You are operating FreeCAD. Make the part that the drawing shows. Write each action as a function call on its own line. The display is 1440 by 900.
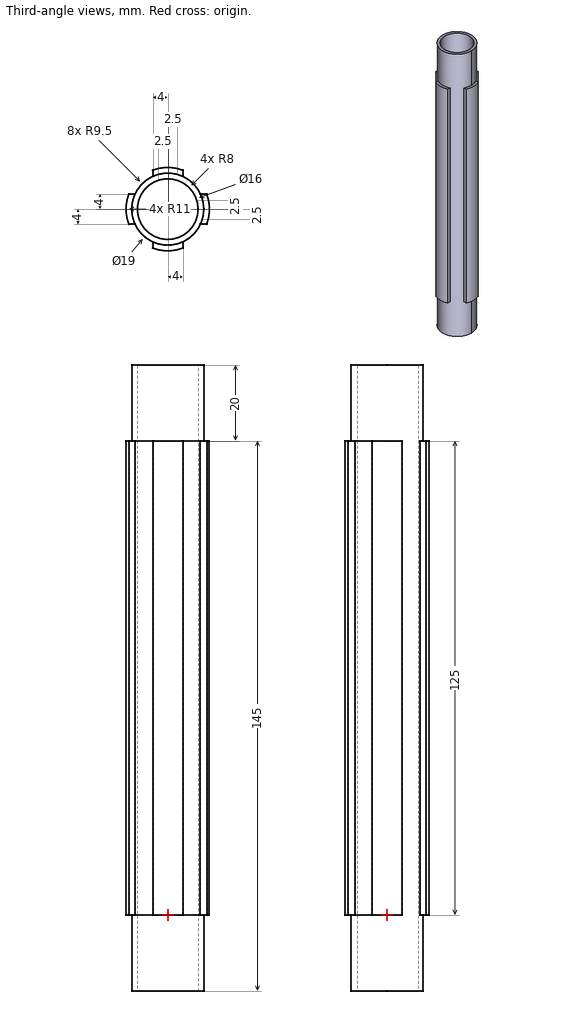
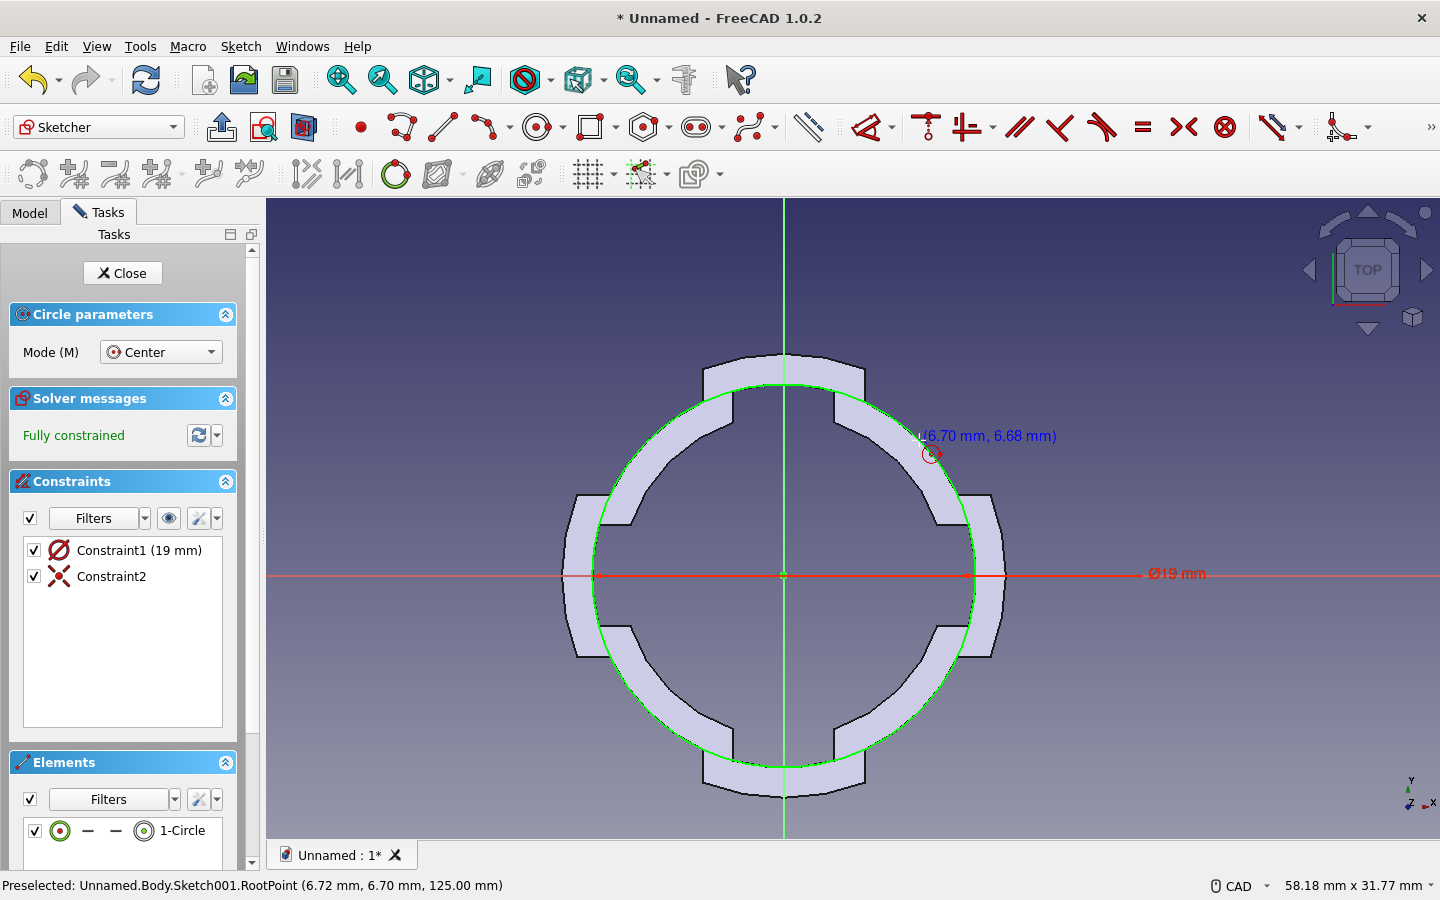
click(784, 576)
move(898, 462)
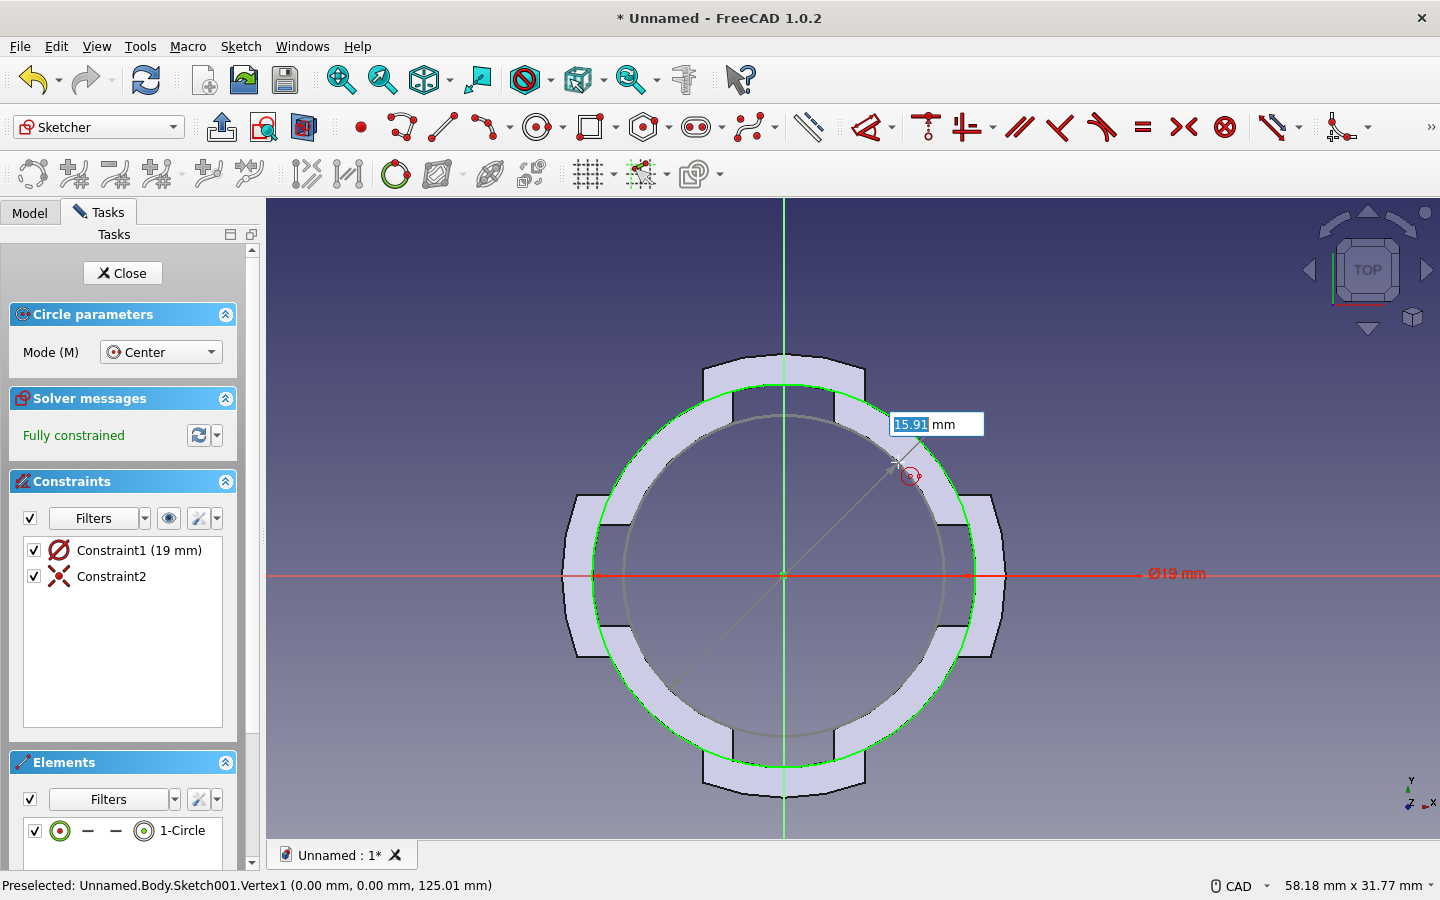
text(16)
key(Return)
key(Escape)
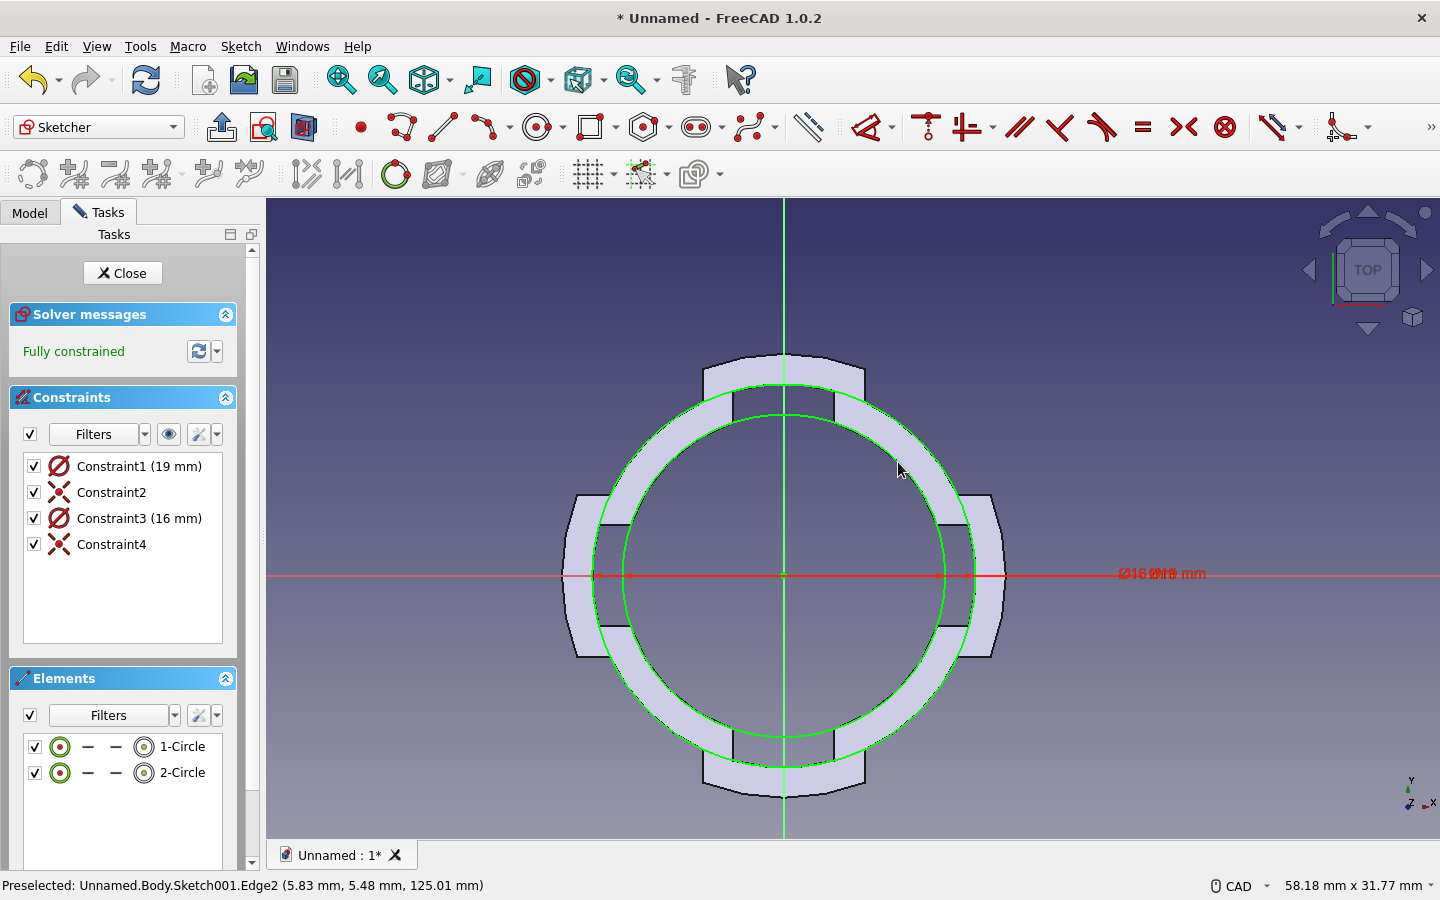
click(123, 273)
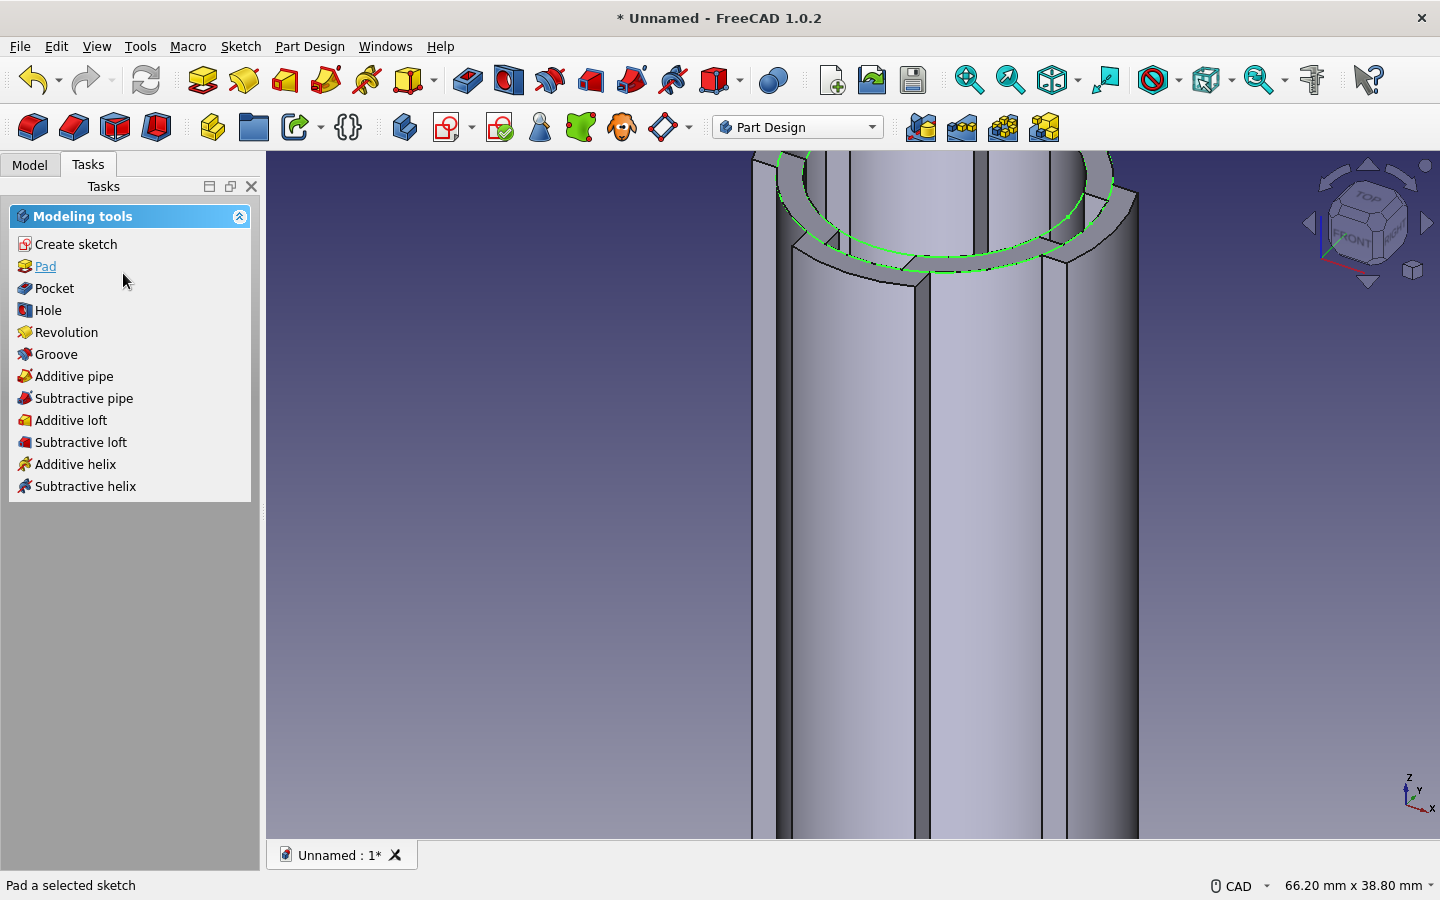
click(203, 80)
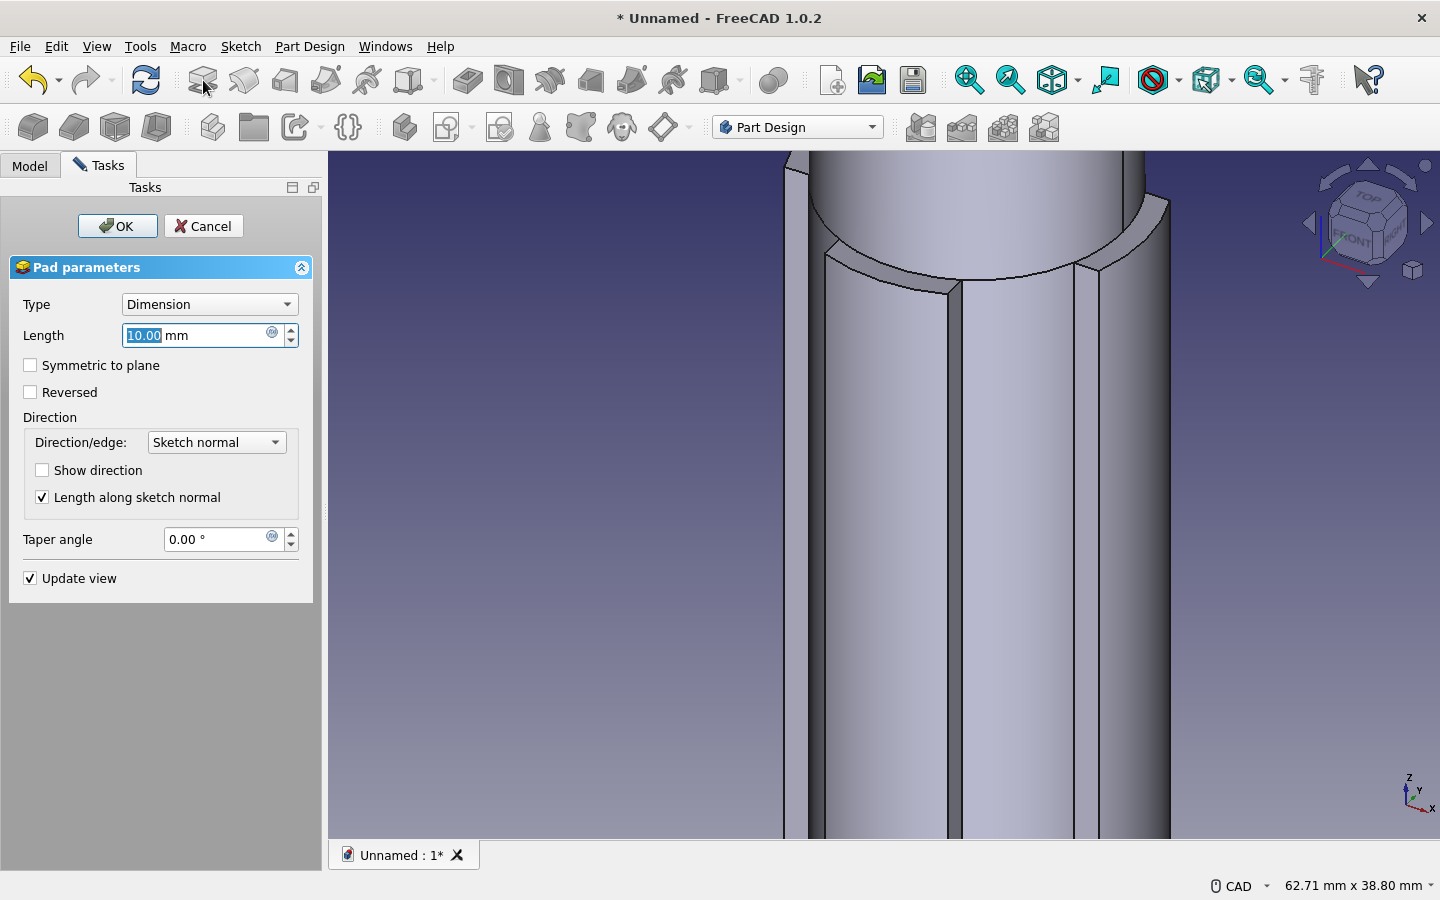
click(210, 304)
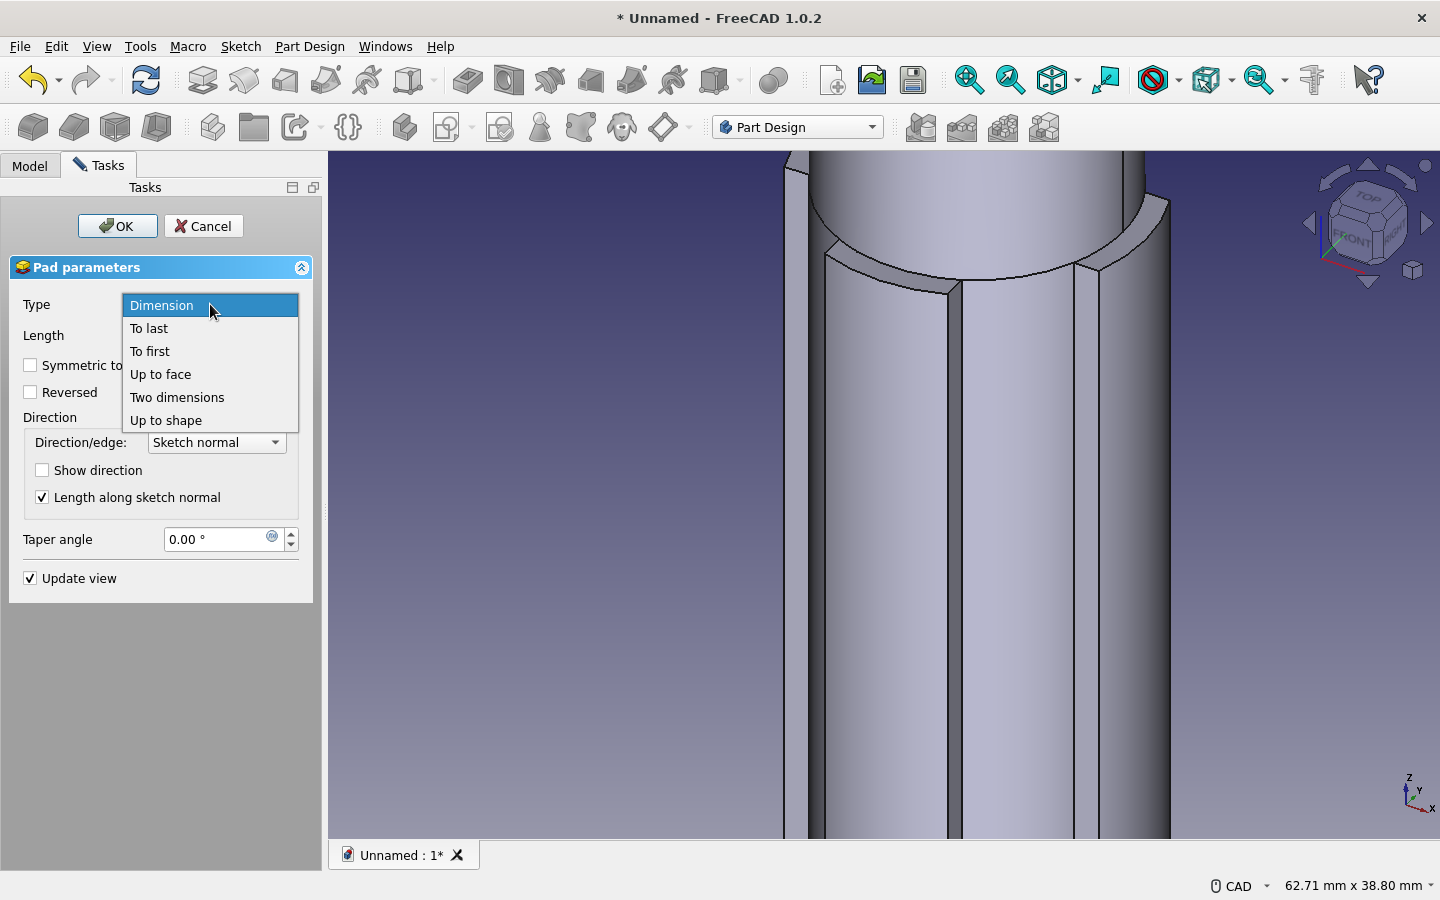
click(208, 398)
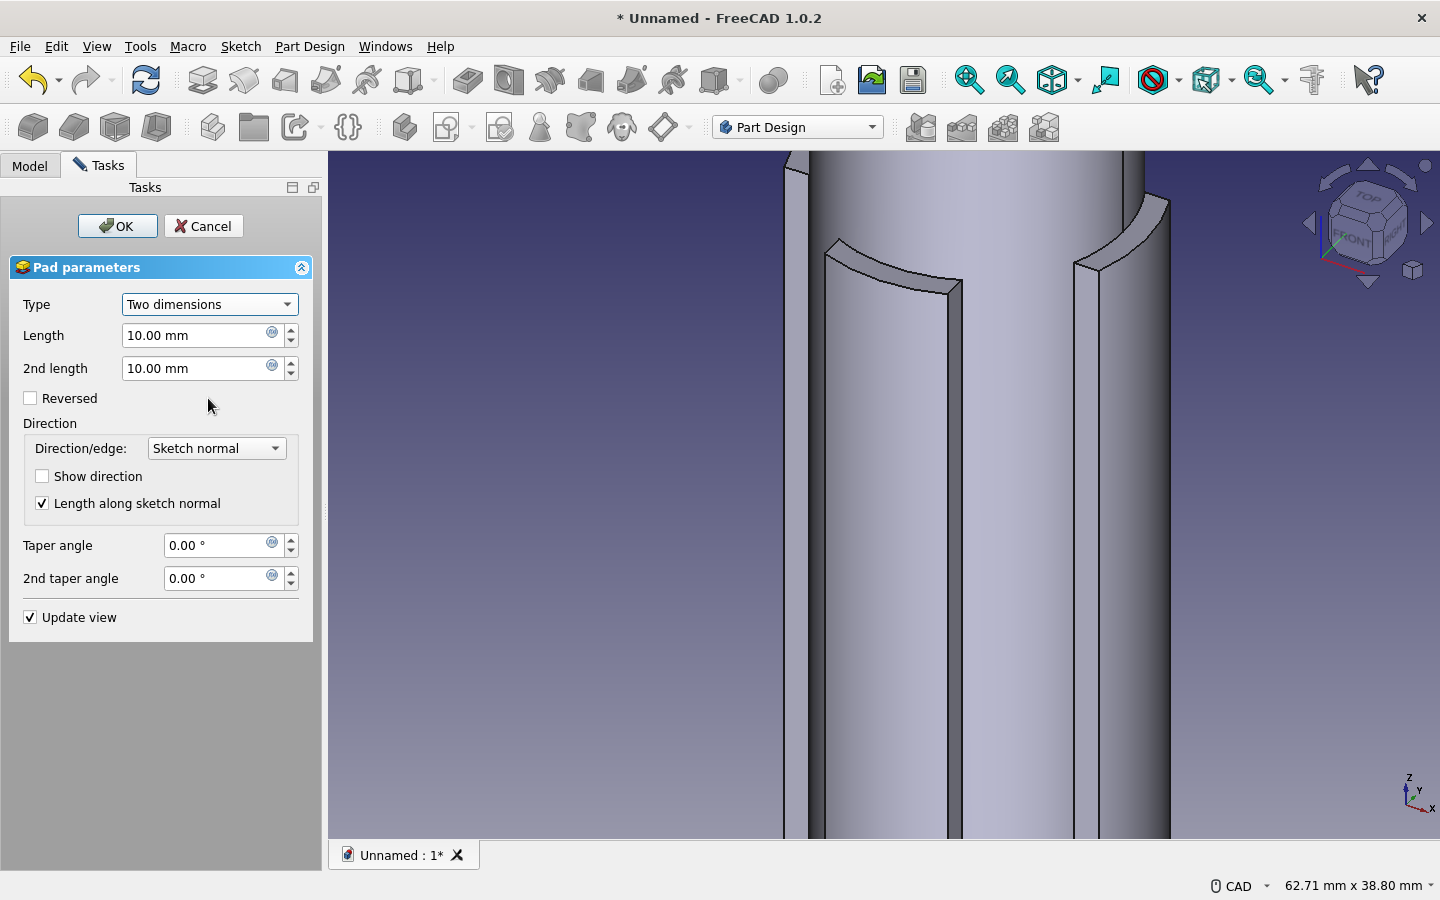
triple_click(204, 336)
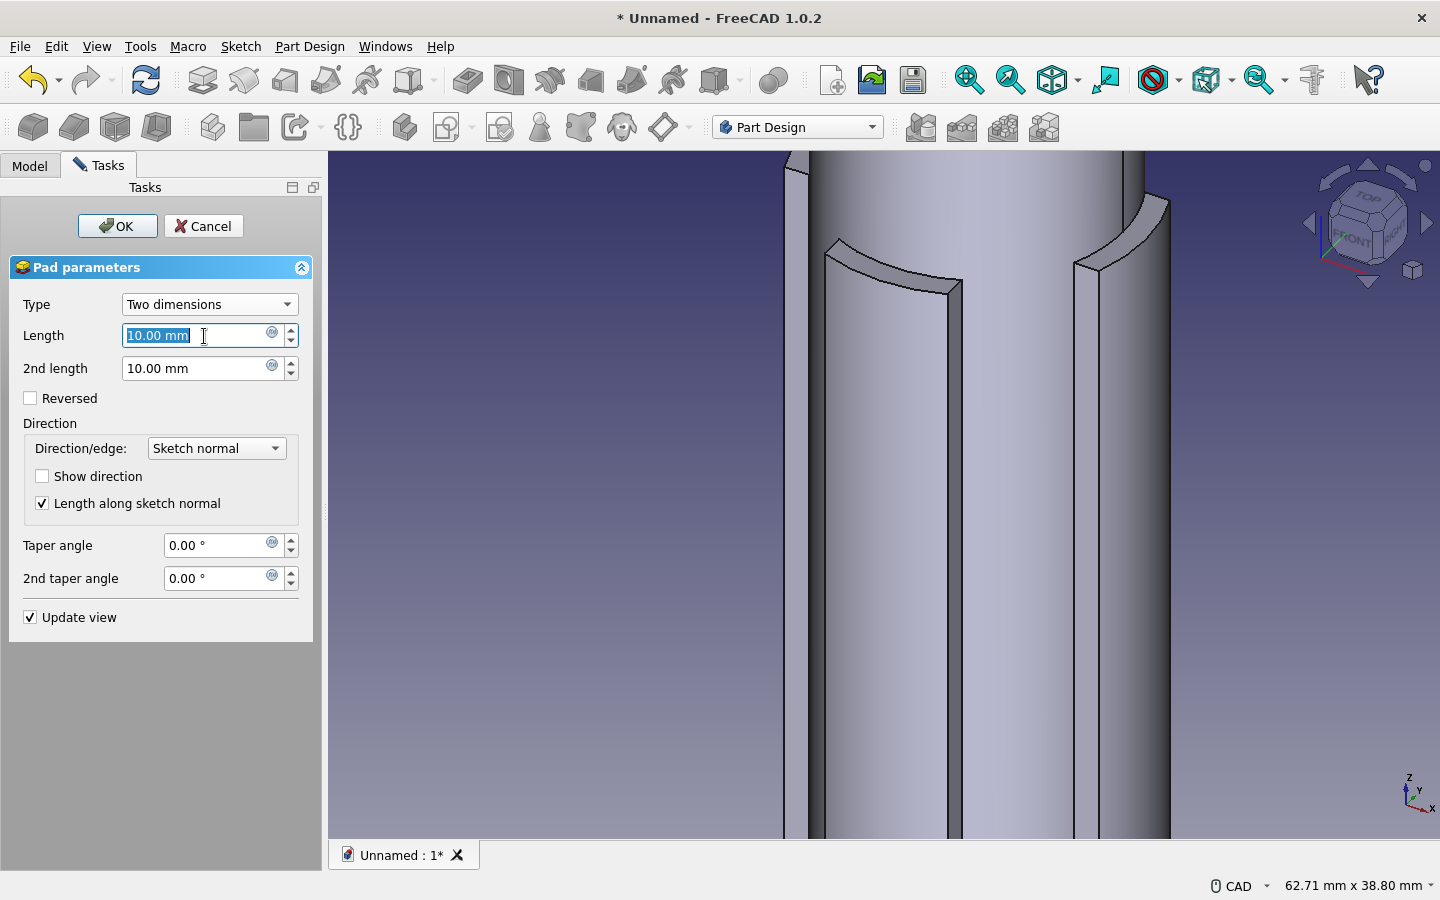
text(20)
key(Tab)